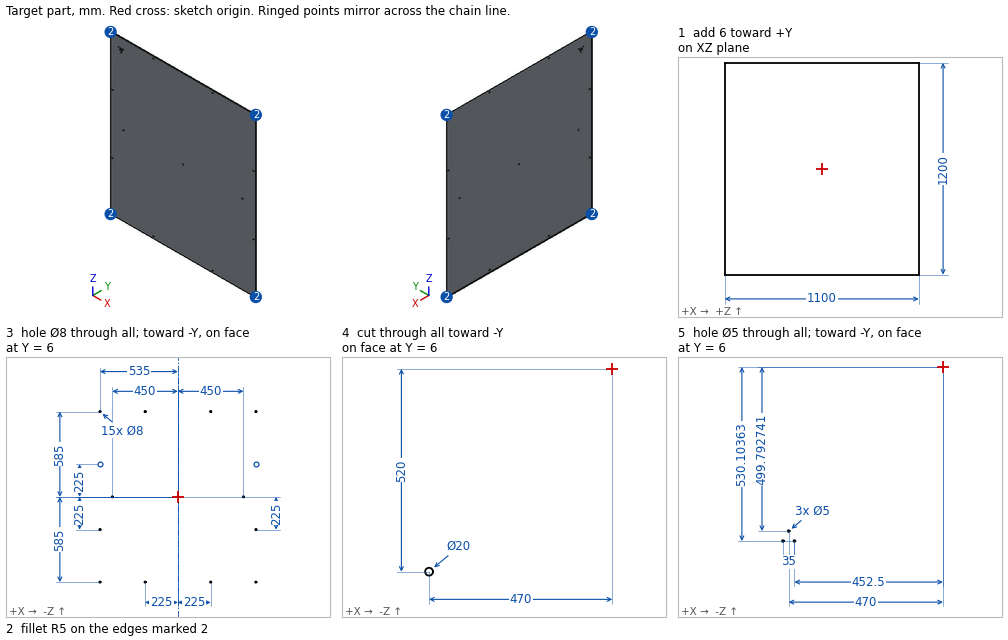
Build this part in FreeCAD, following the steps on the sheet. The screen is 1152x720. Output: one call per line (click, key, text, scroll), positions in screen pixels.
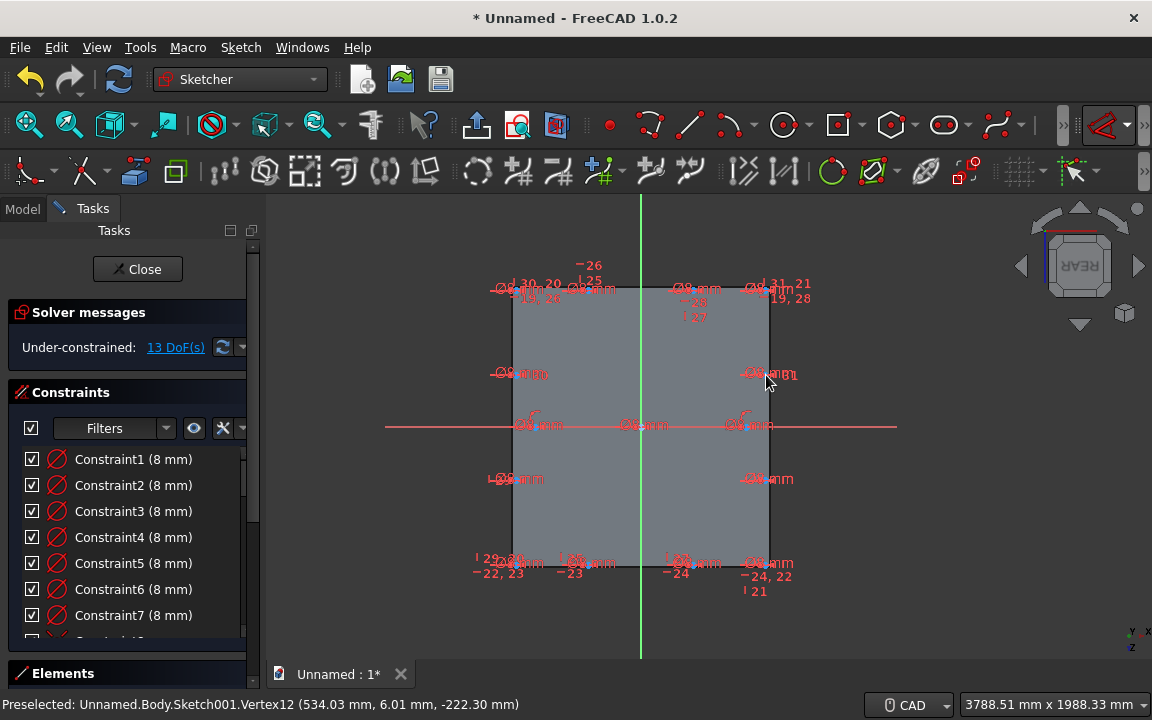
click(766, 565)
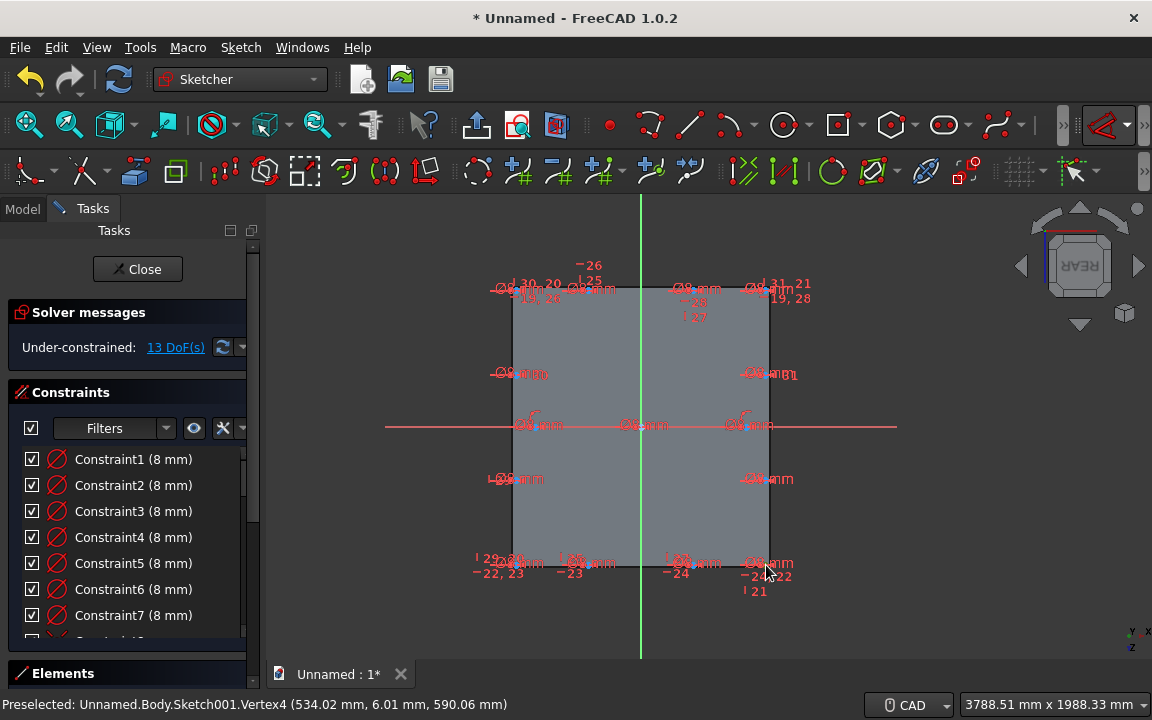
click(766, 481)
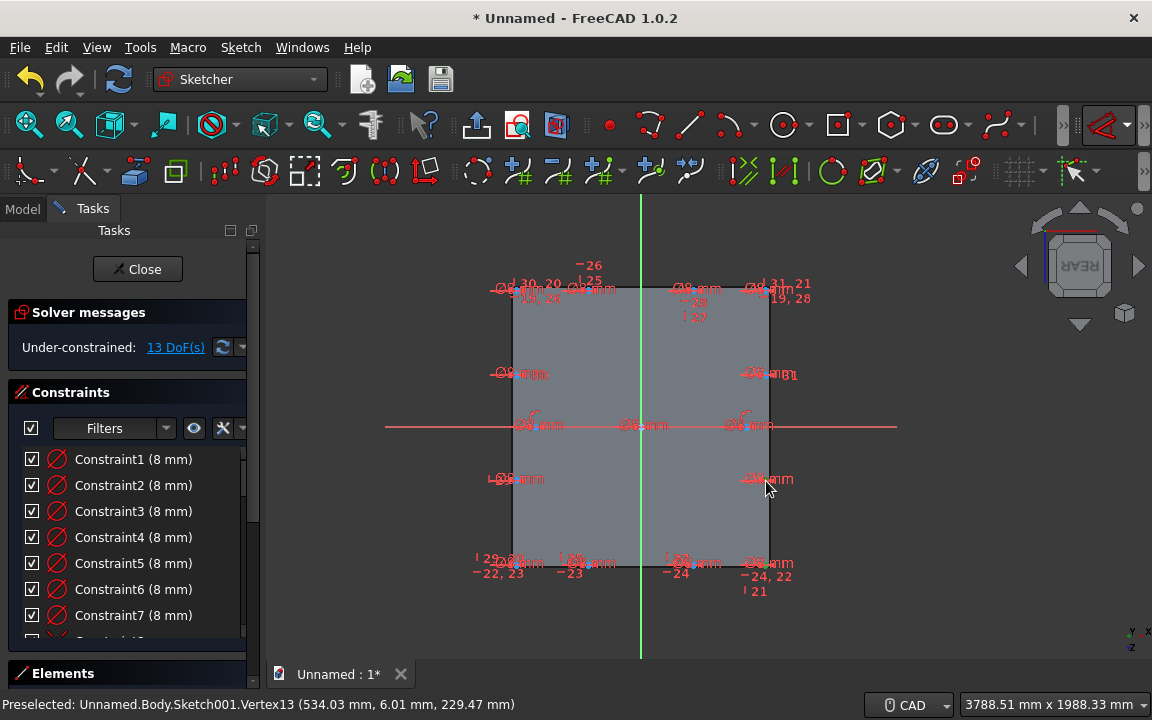
key(v)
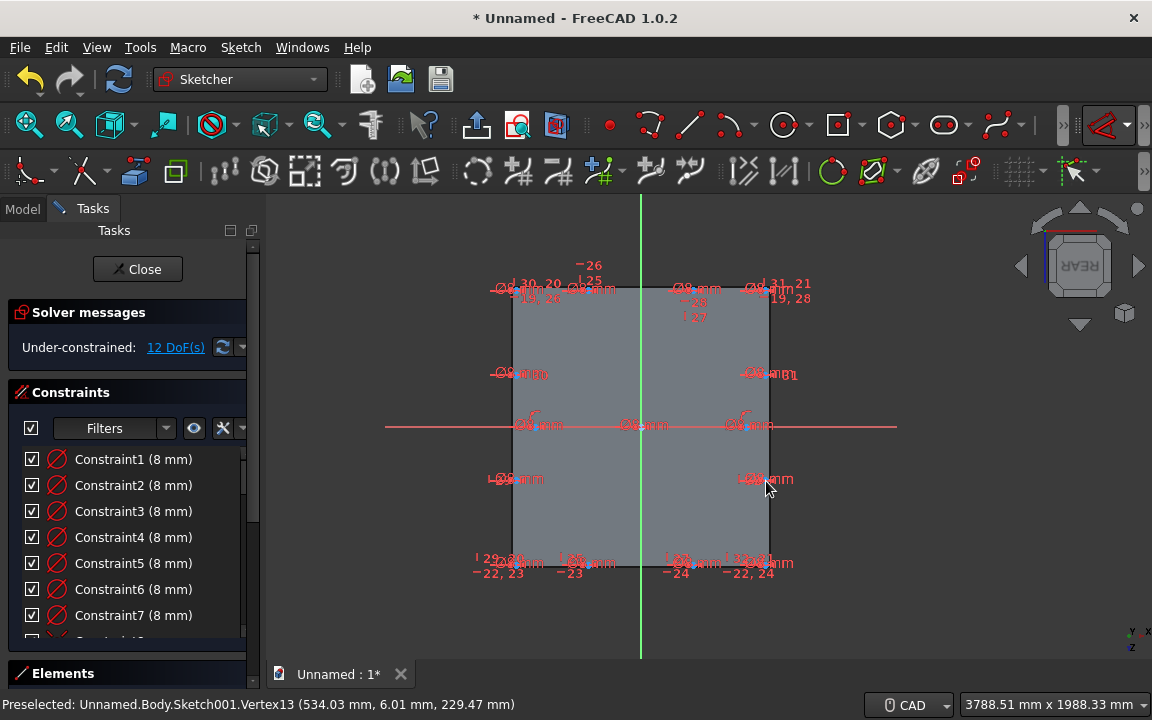
click(516, 375)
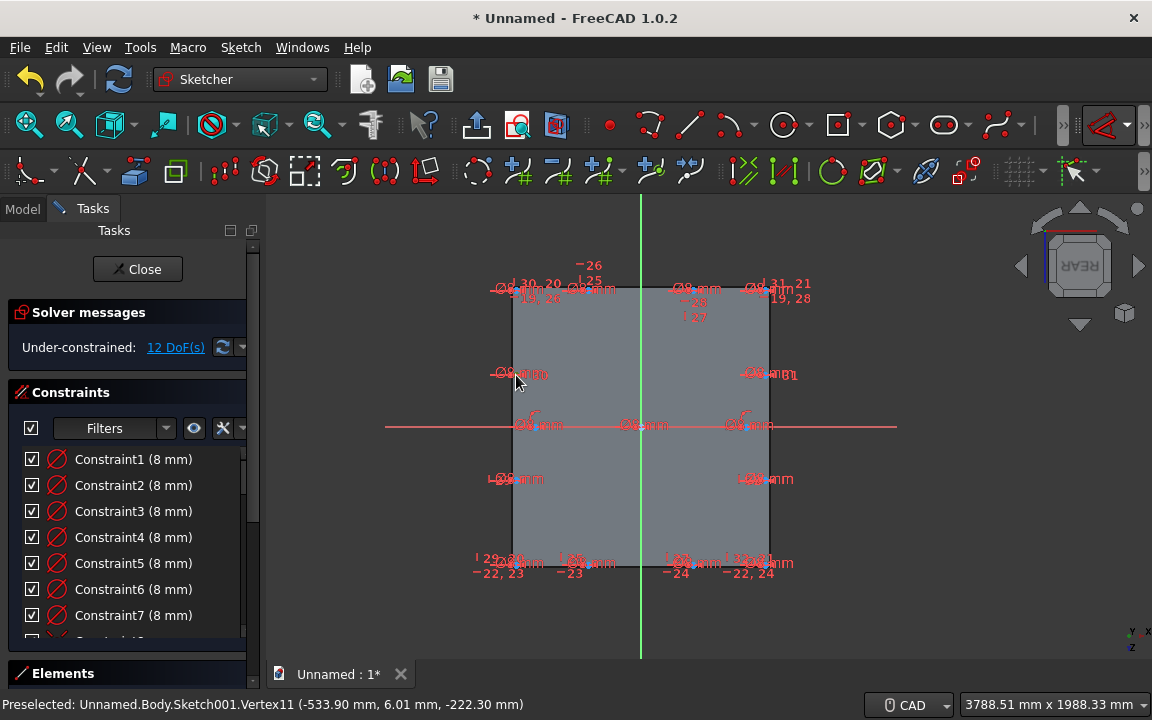
click(766, 375)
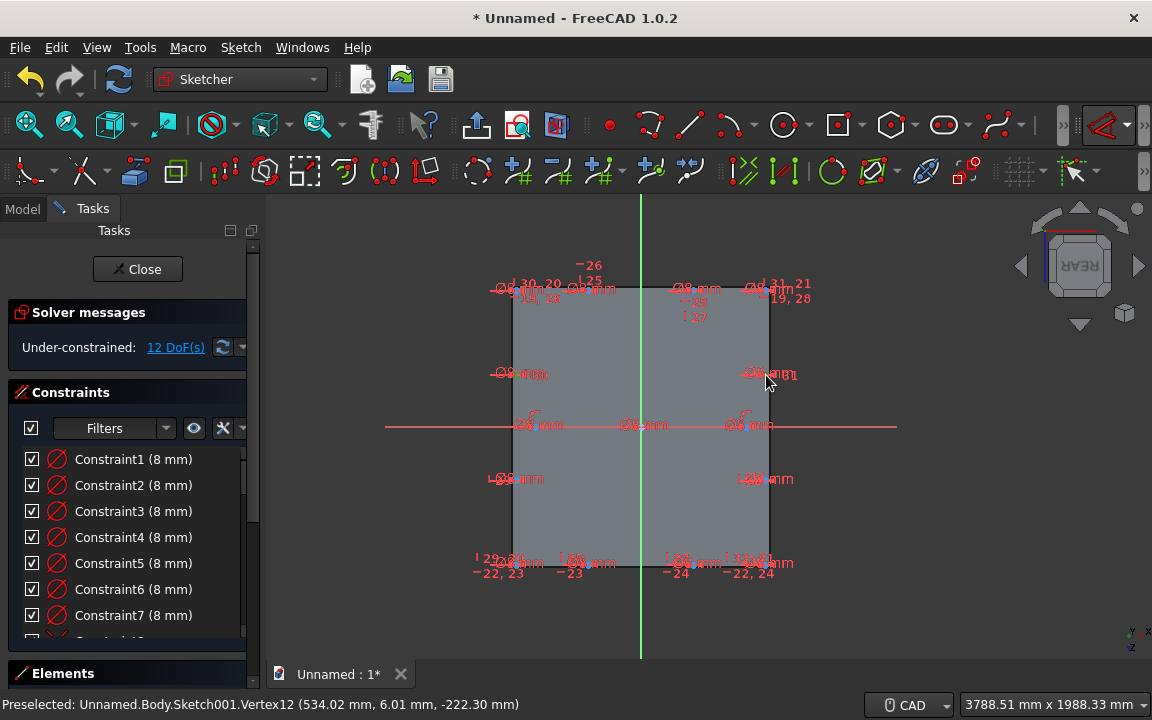
click(641, 602)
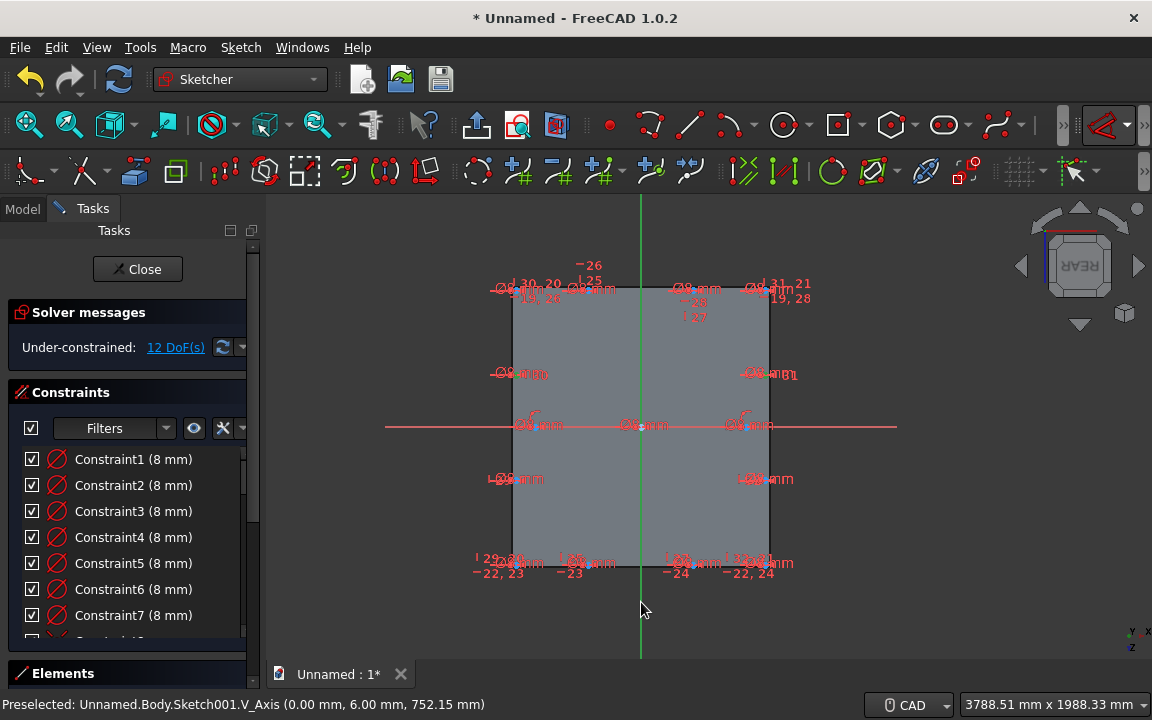
key(s)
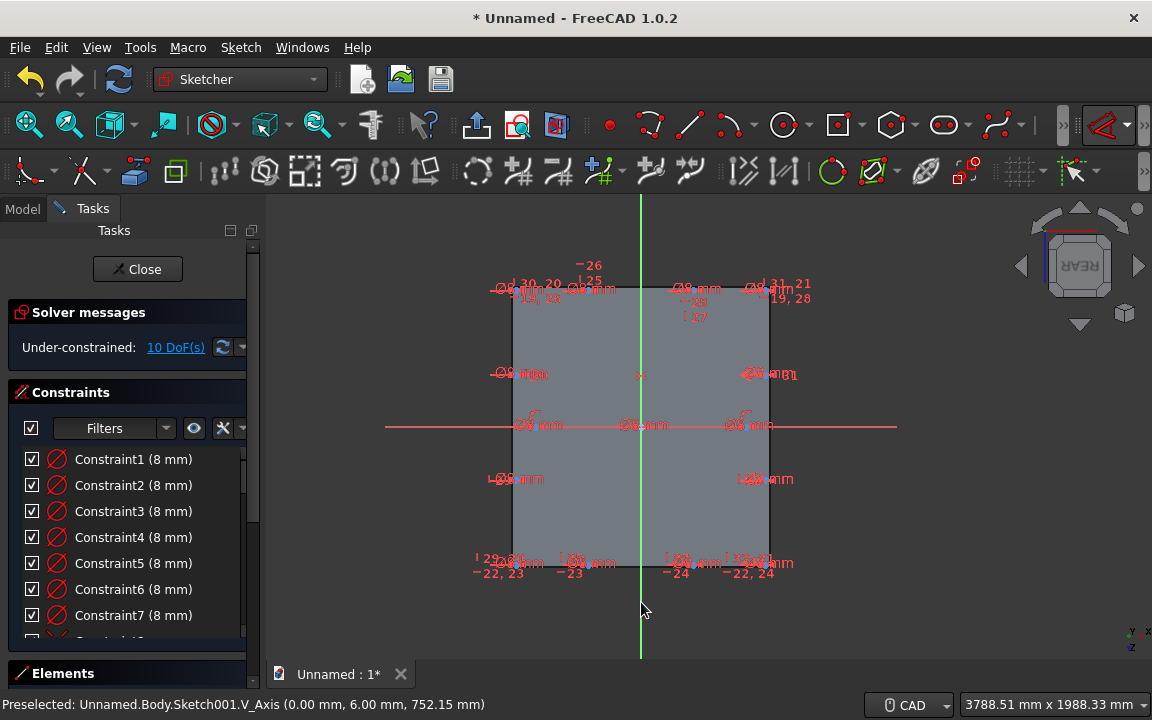
click(516, 291)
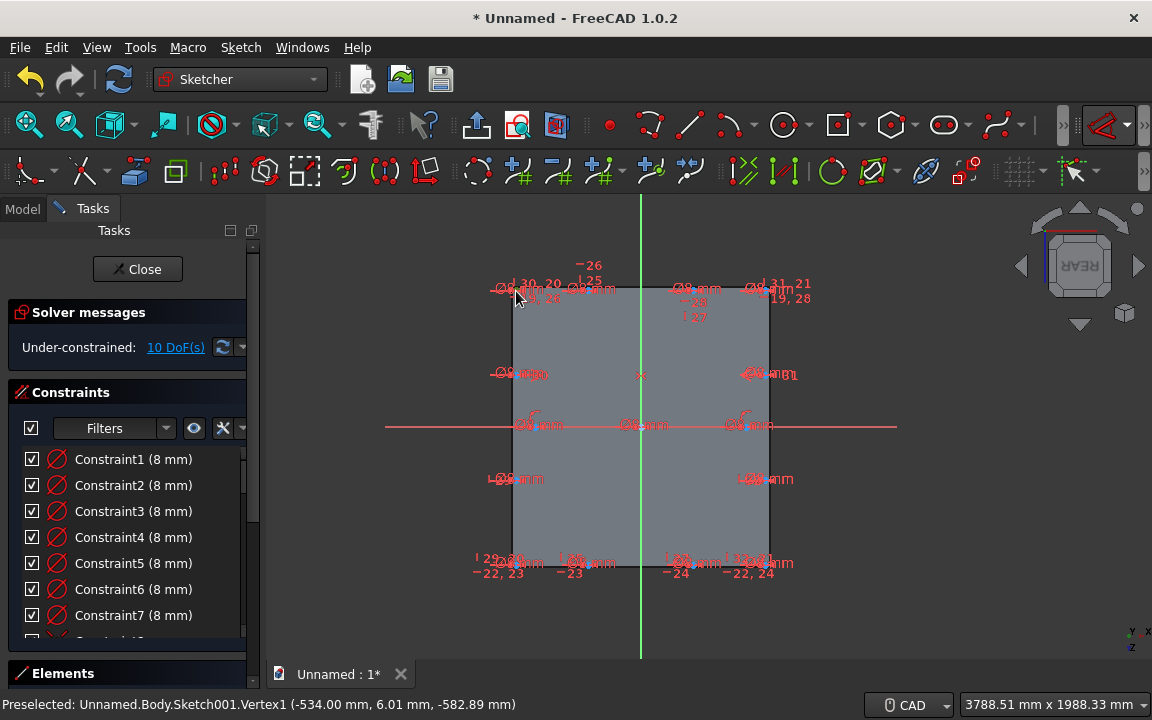
click(1130, 126)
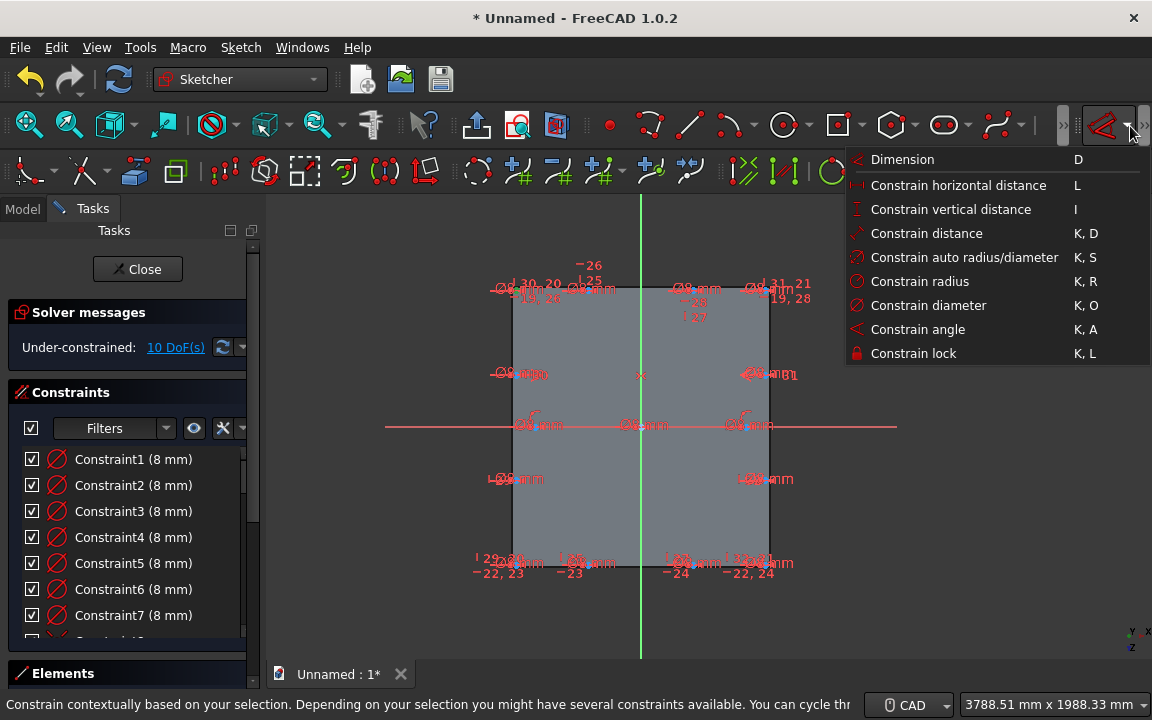
click(998, 185)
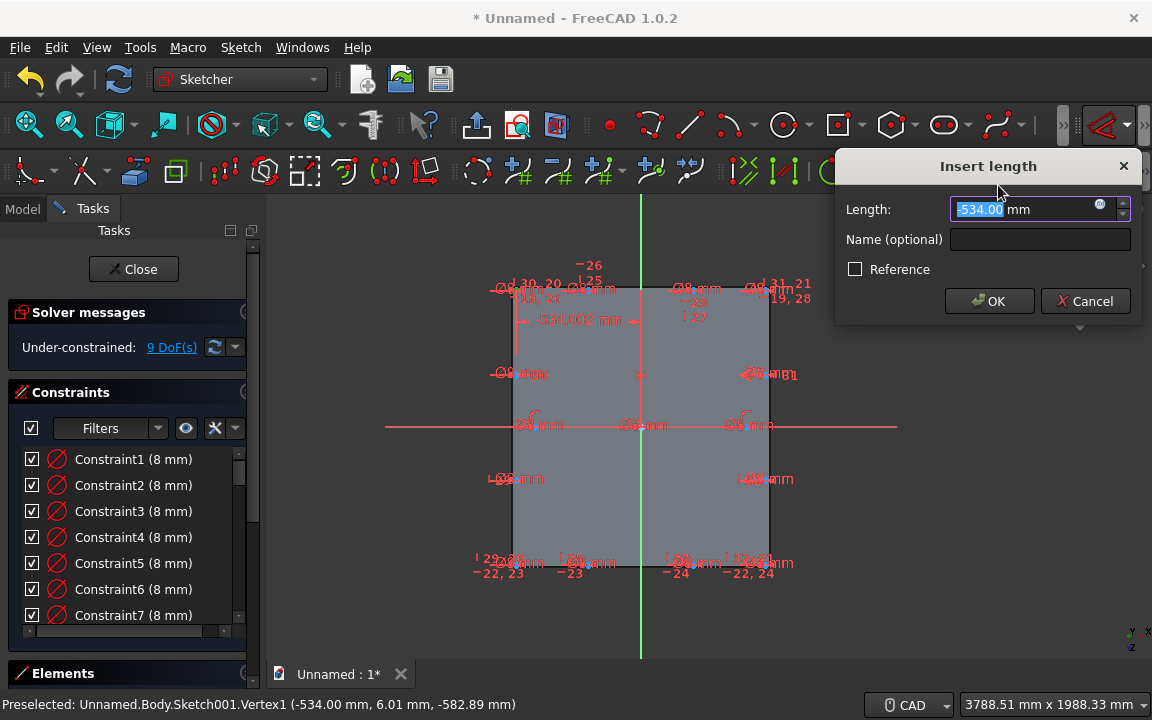
text(-535)
key(Return)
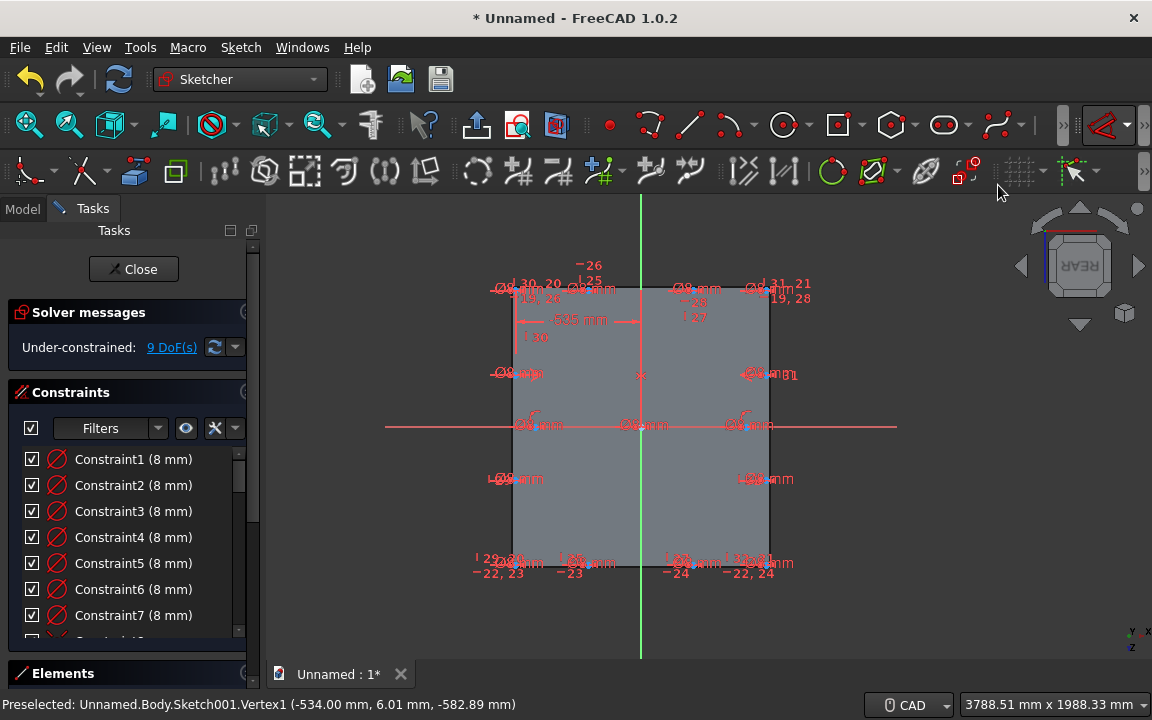
click(516, 291)